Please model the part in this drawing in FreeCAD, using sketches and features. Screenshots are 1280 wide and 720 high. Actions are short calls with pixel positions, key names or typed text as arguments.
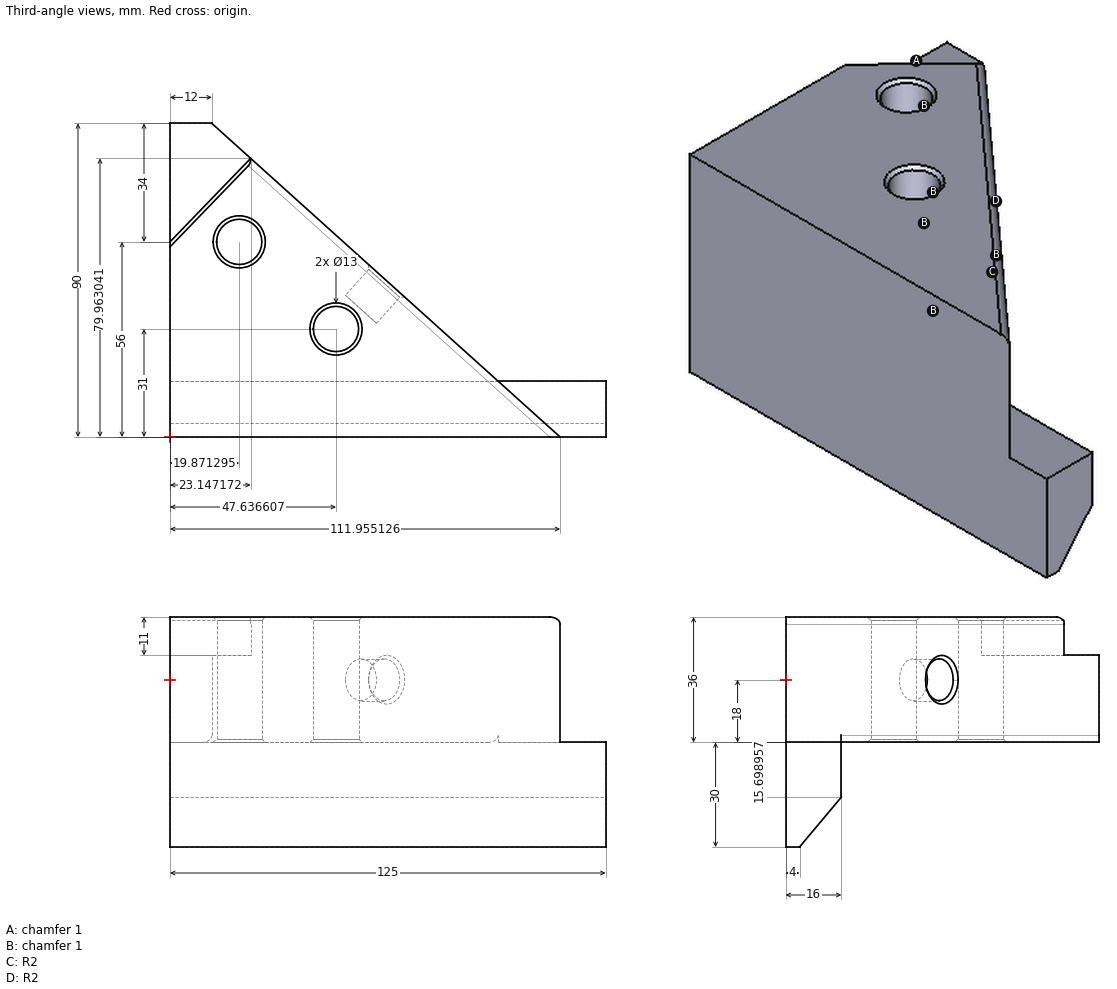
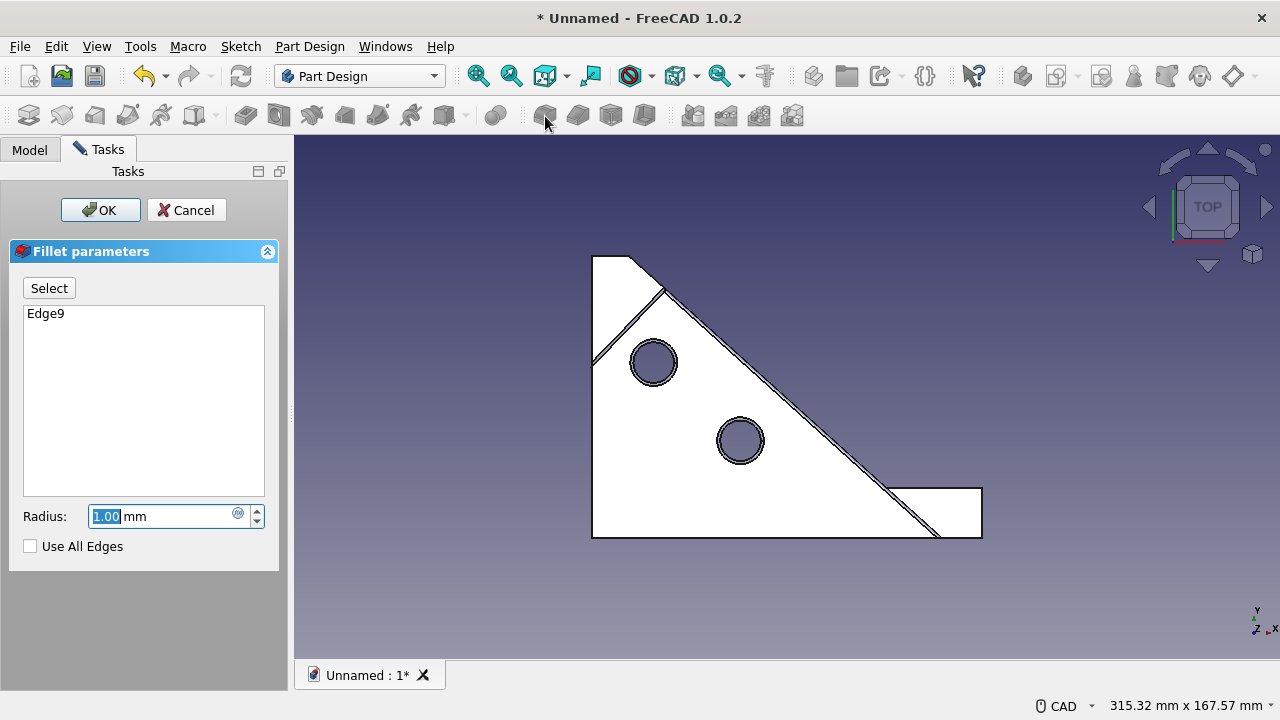
text(2)
key(Tab)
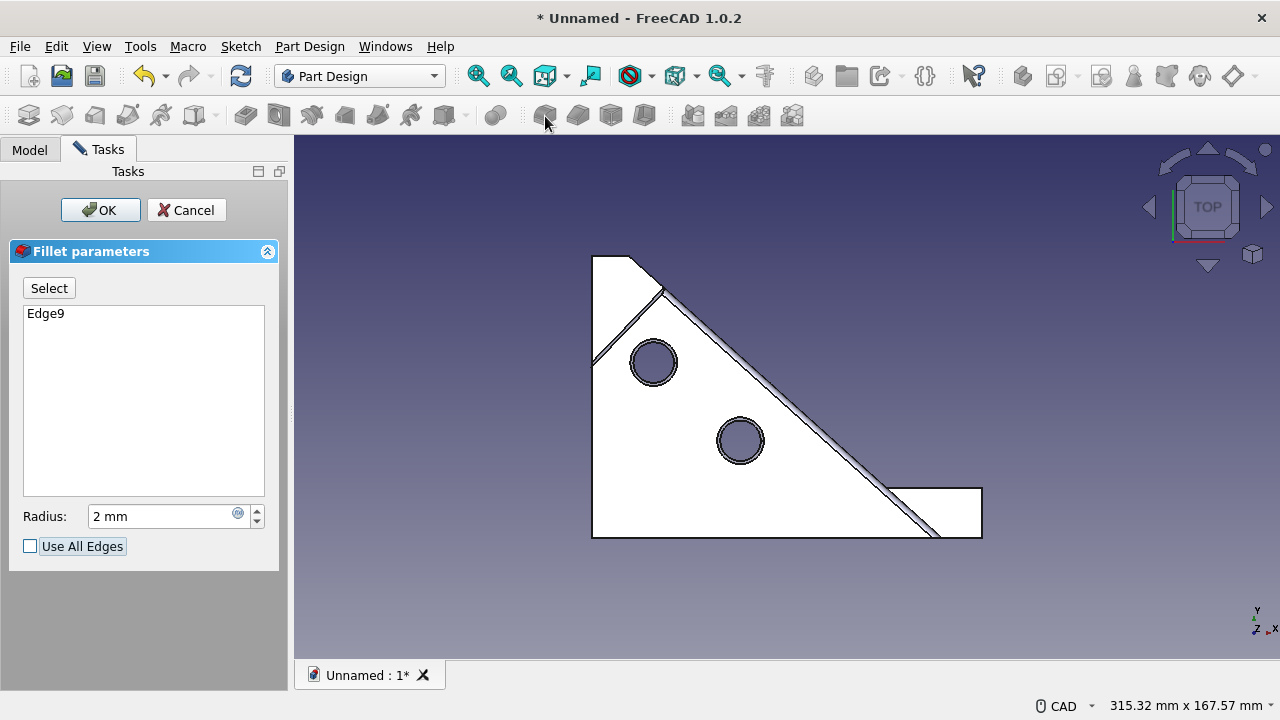
click(101, 210)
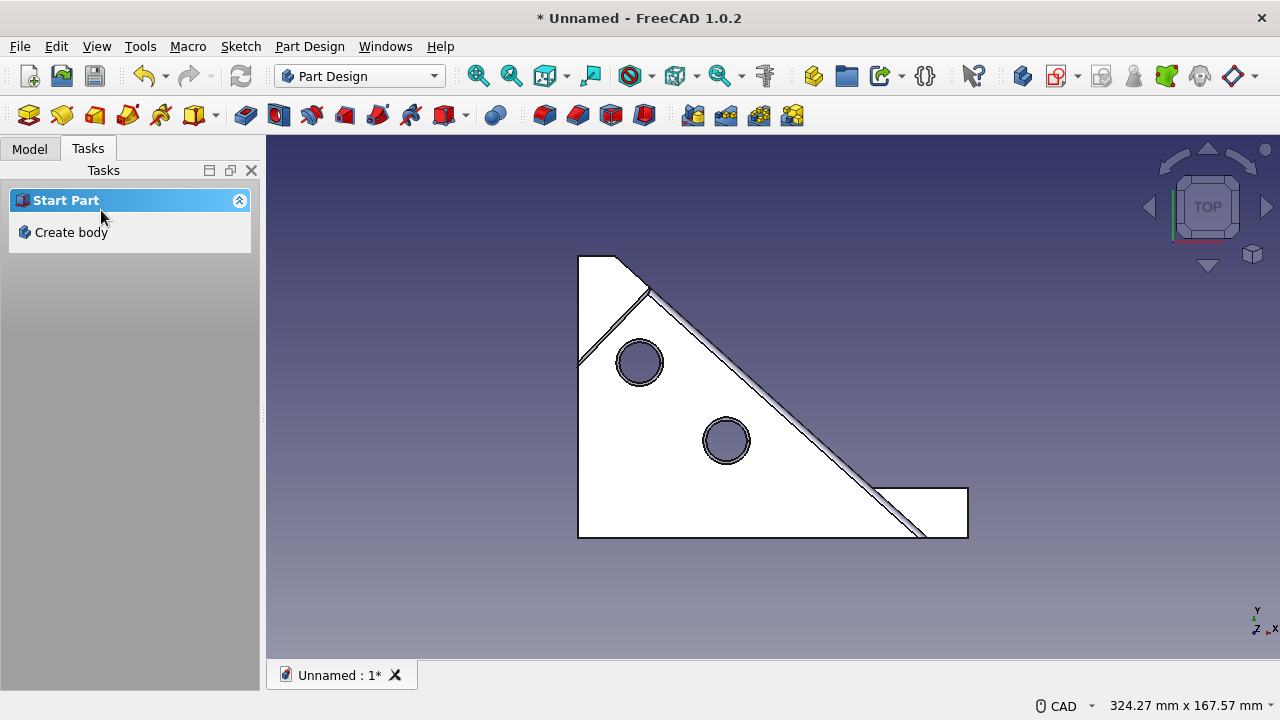
key(0)